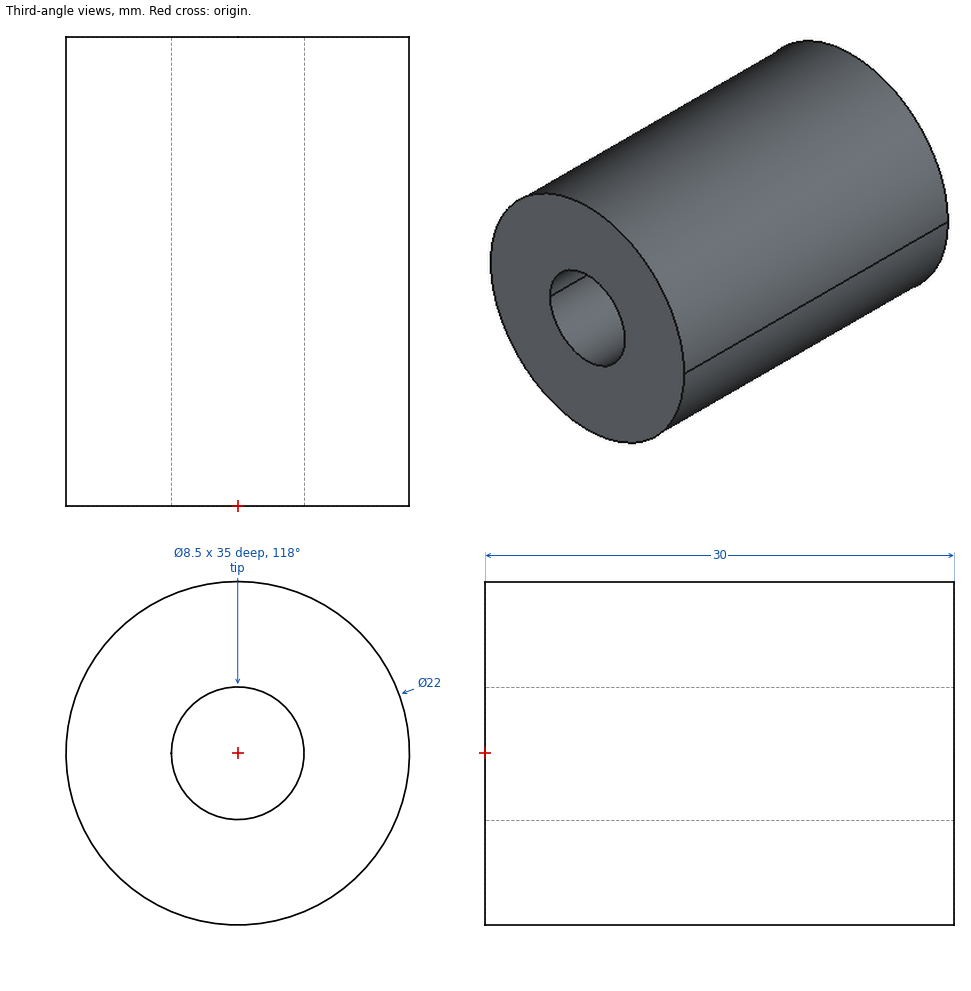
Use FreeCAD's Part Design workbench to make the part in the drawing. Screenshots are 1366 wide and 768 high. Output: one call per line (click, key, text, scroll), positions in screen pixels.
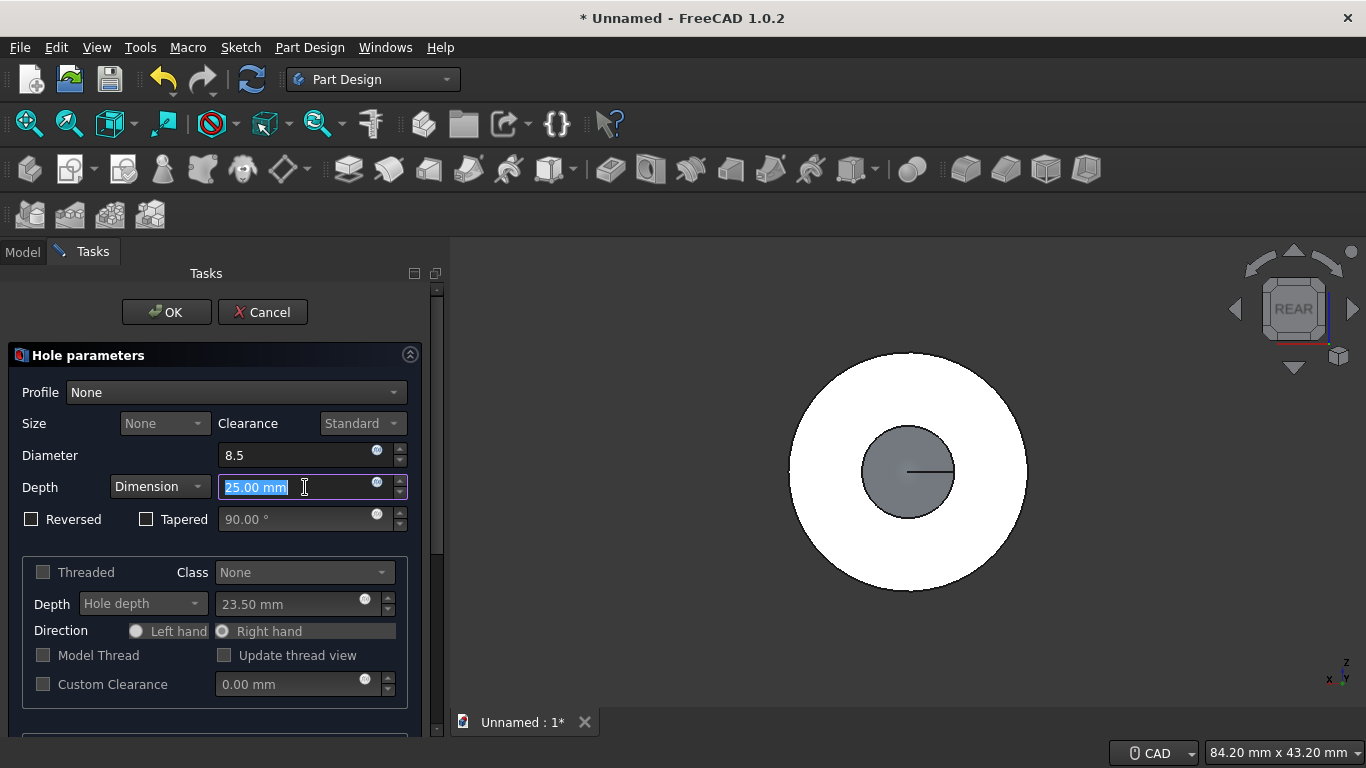
text(35)
key(Tab)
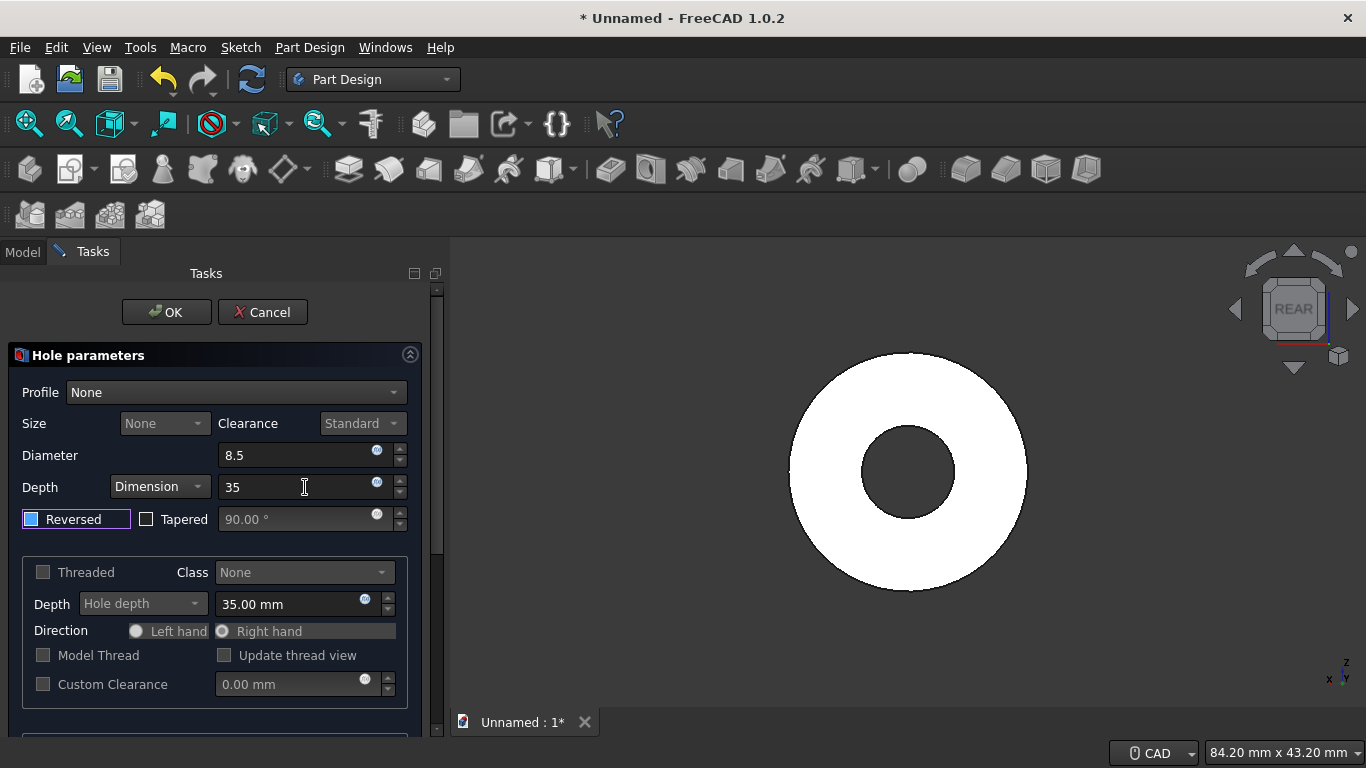
click(167, 312)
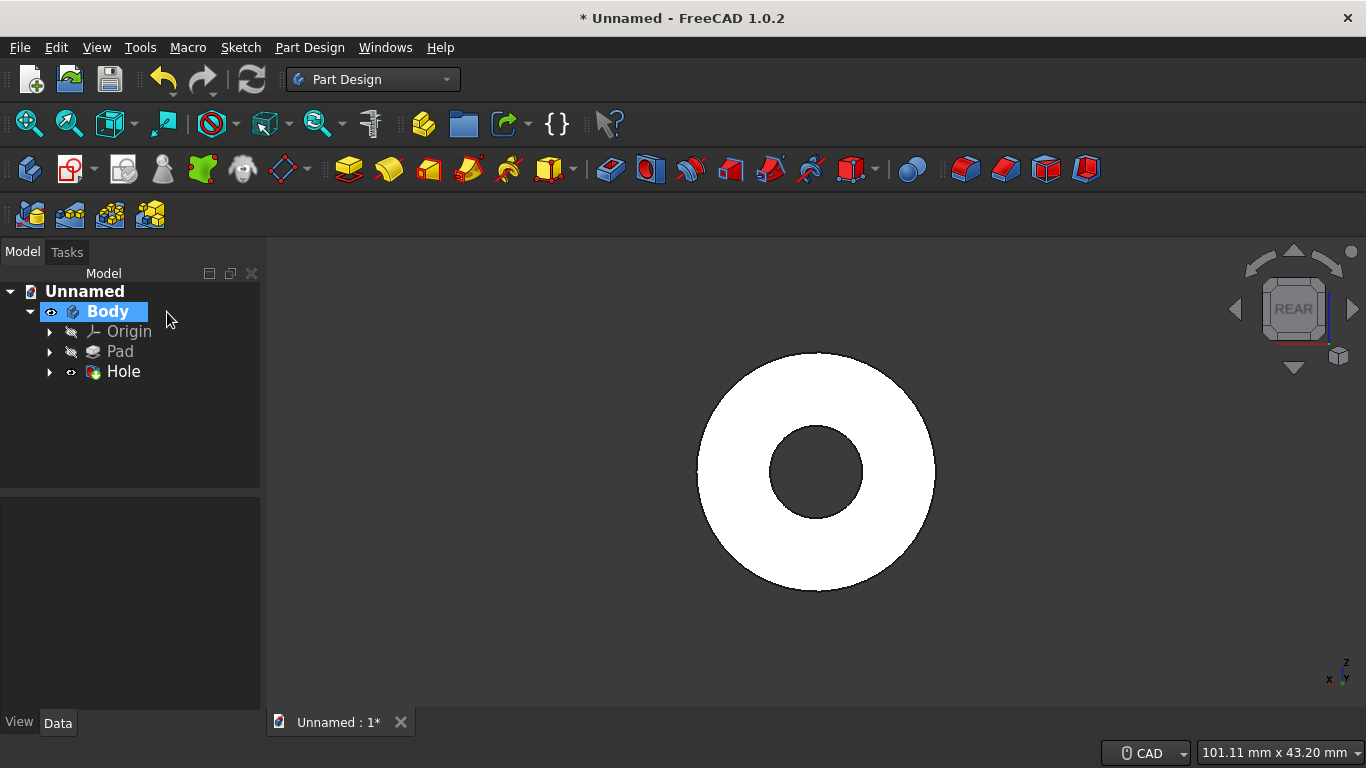
key(0)